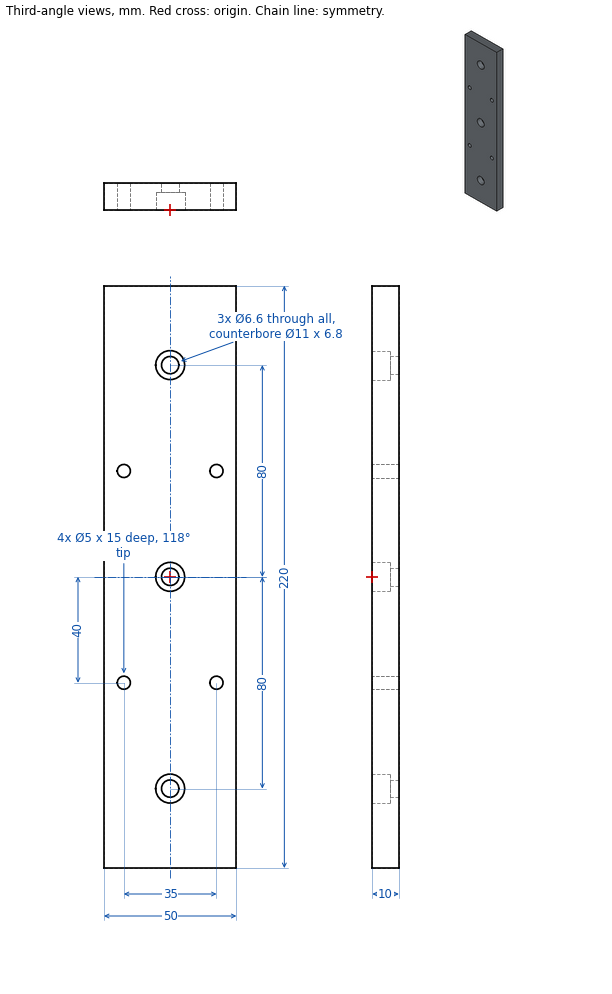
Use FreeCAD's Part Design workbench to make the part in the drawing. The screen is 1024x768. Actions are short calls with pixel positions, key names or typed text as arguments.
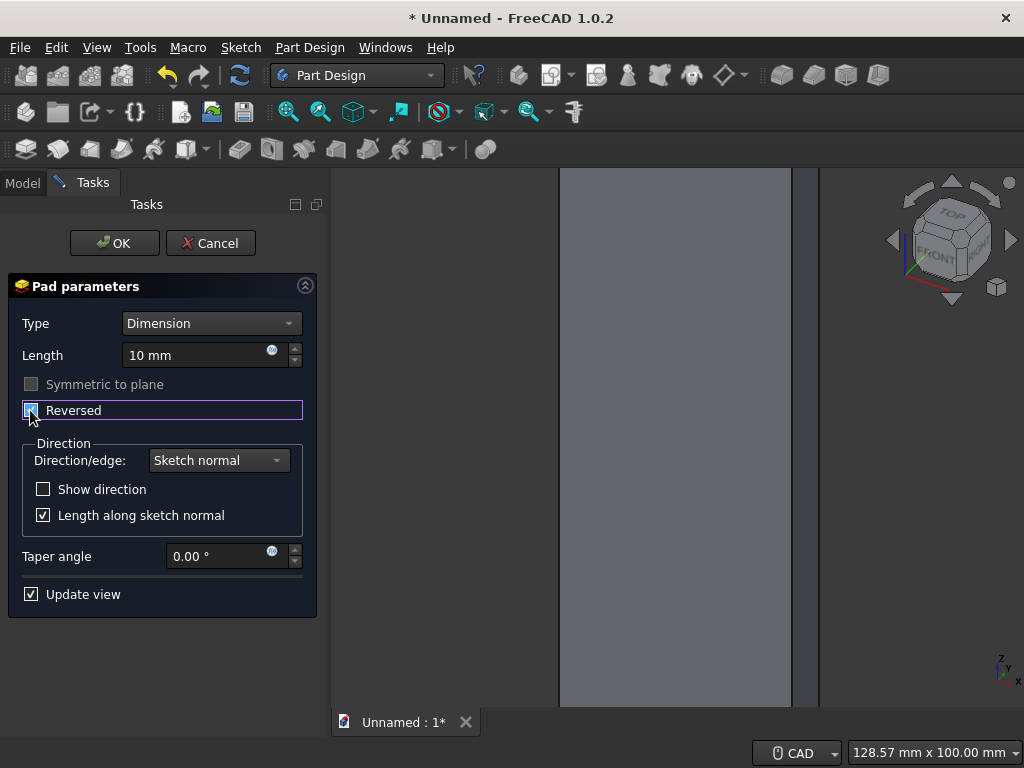
click(115, 243)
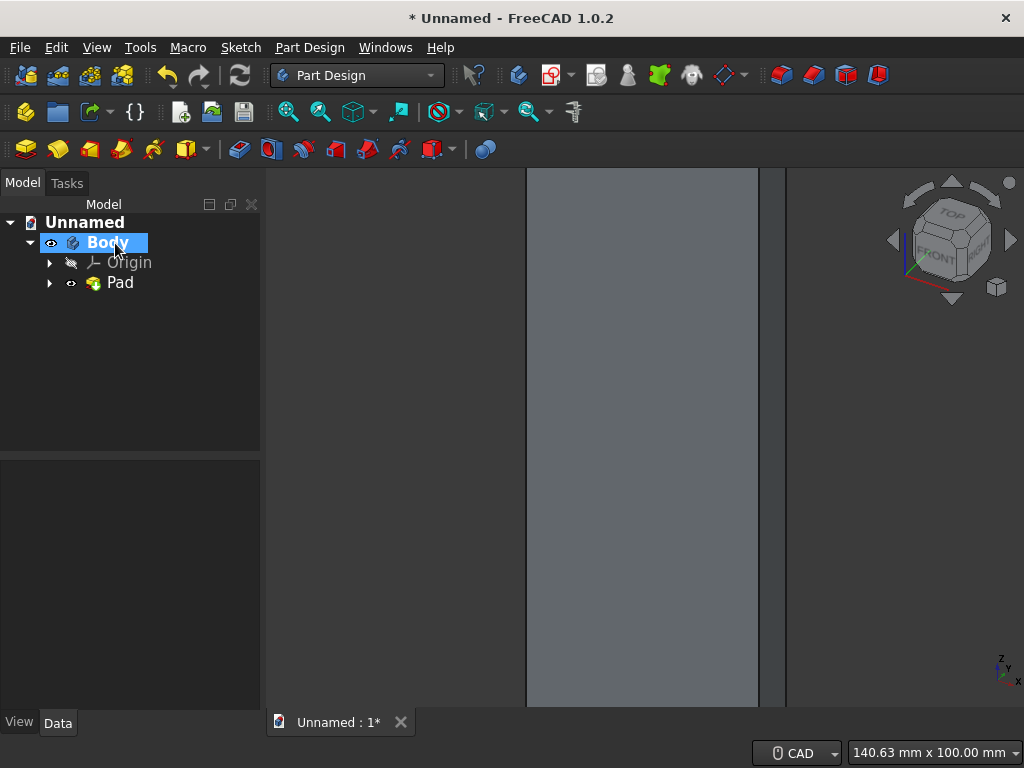
click(290, 112)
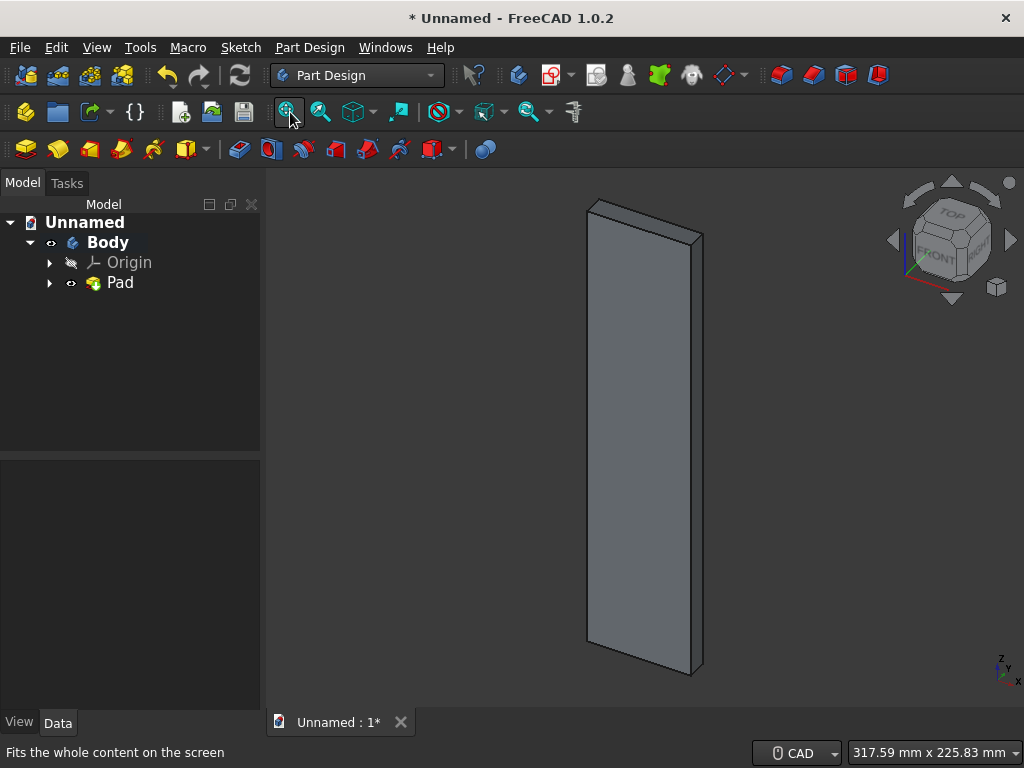
click(552, 76)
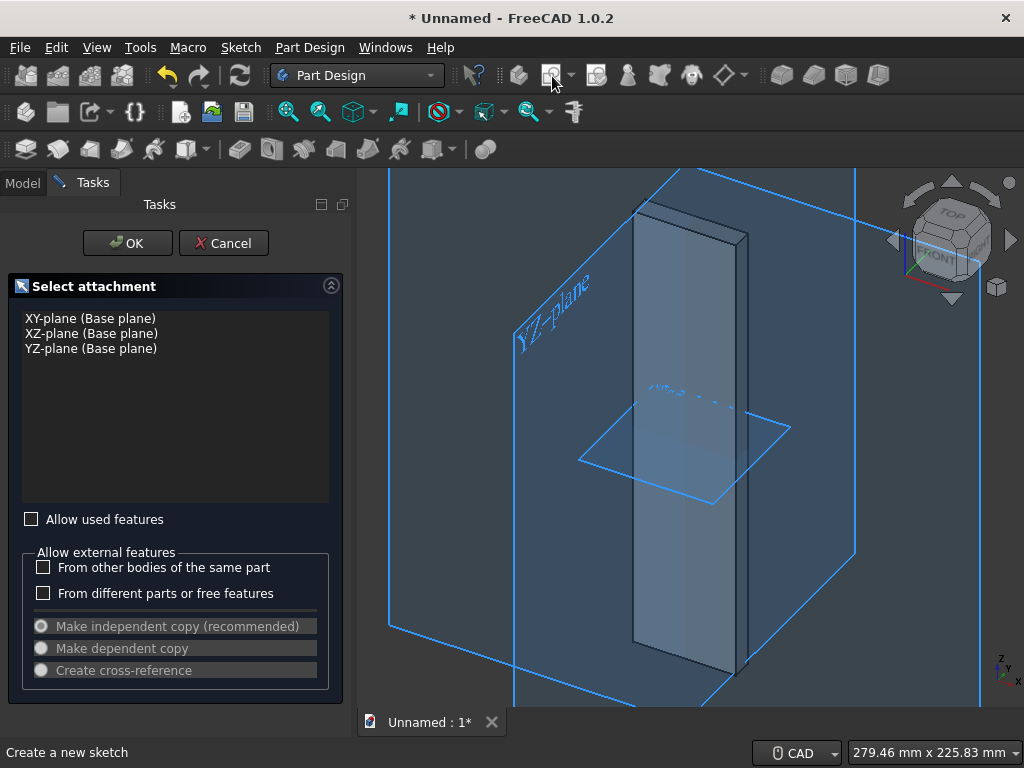
click(82, 334)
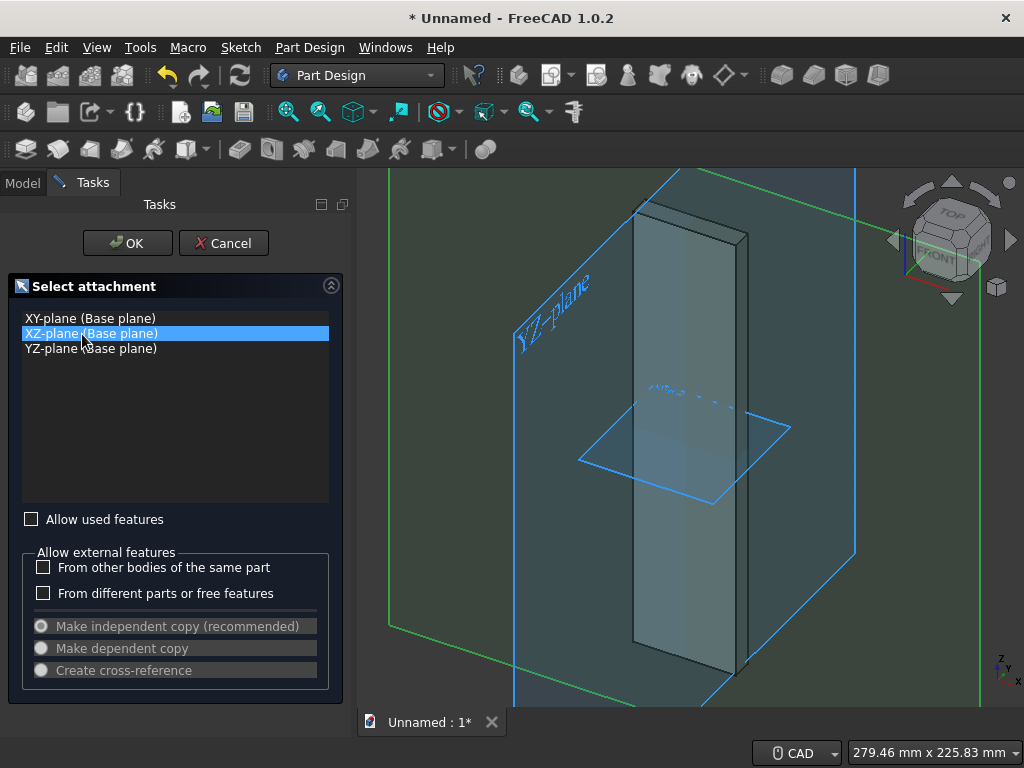
click(128, 243)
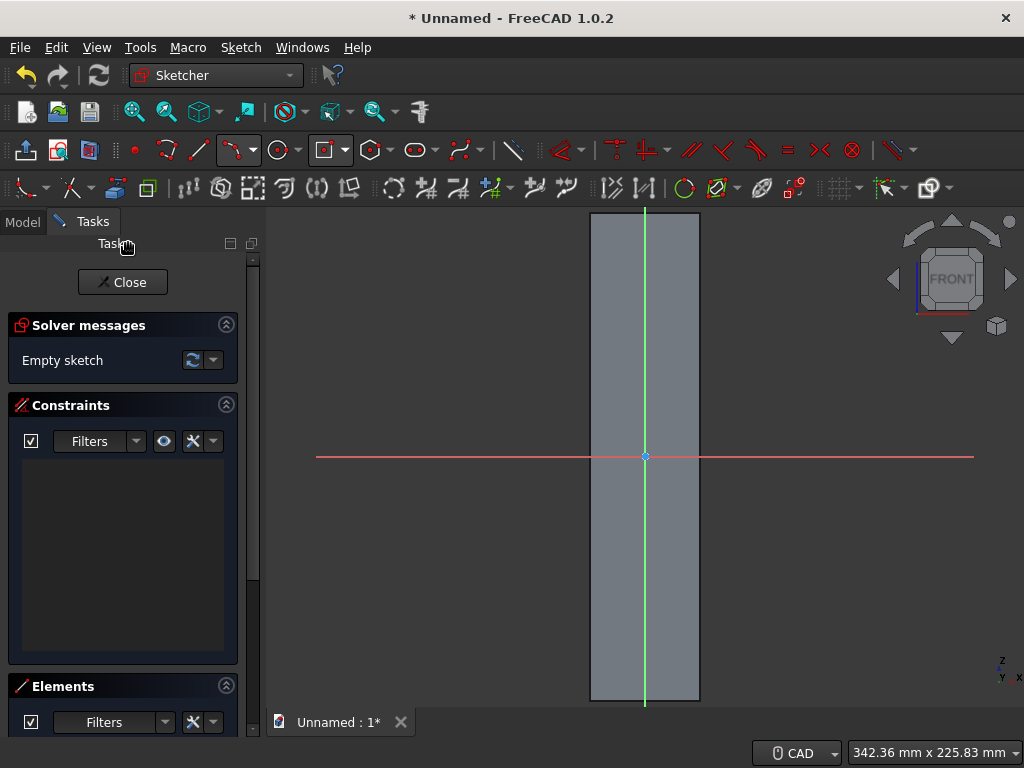
click(278, 150)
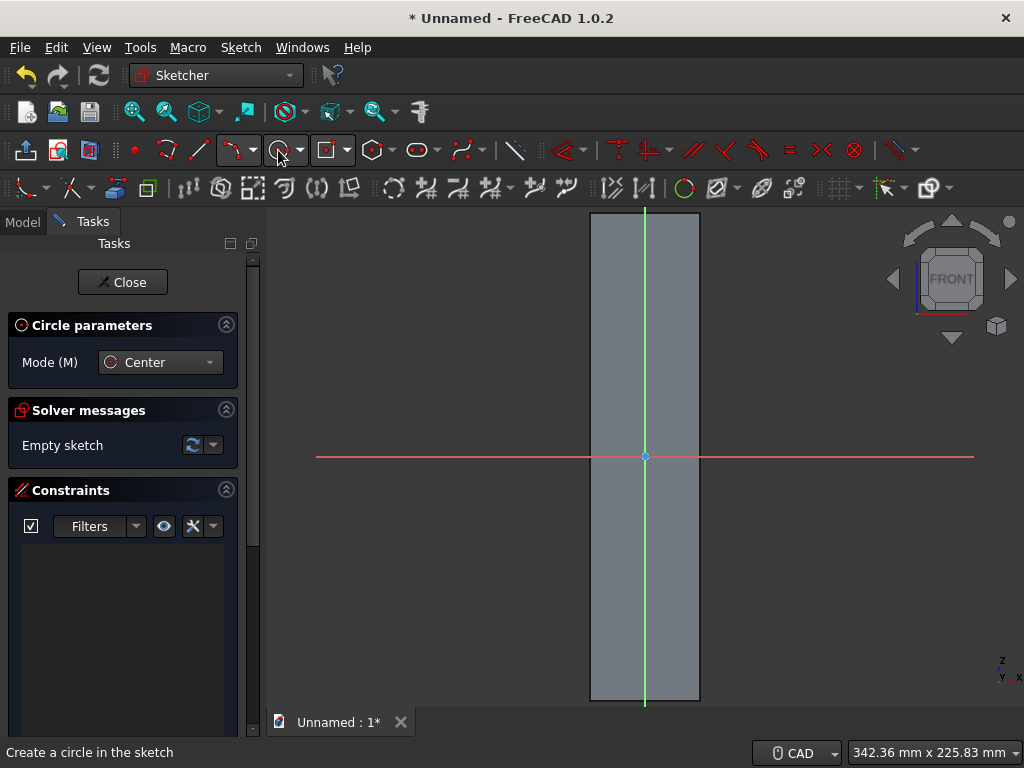
scroll(645, 280, up, 6)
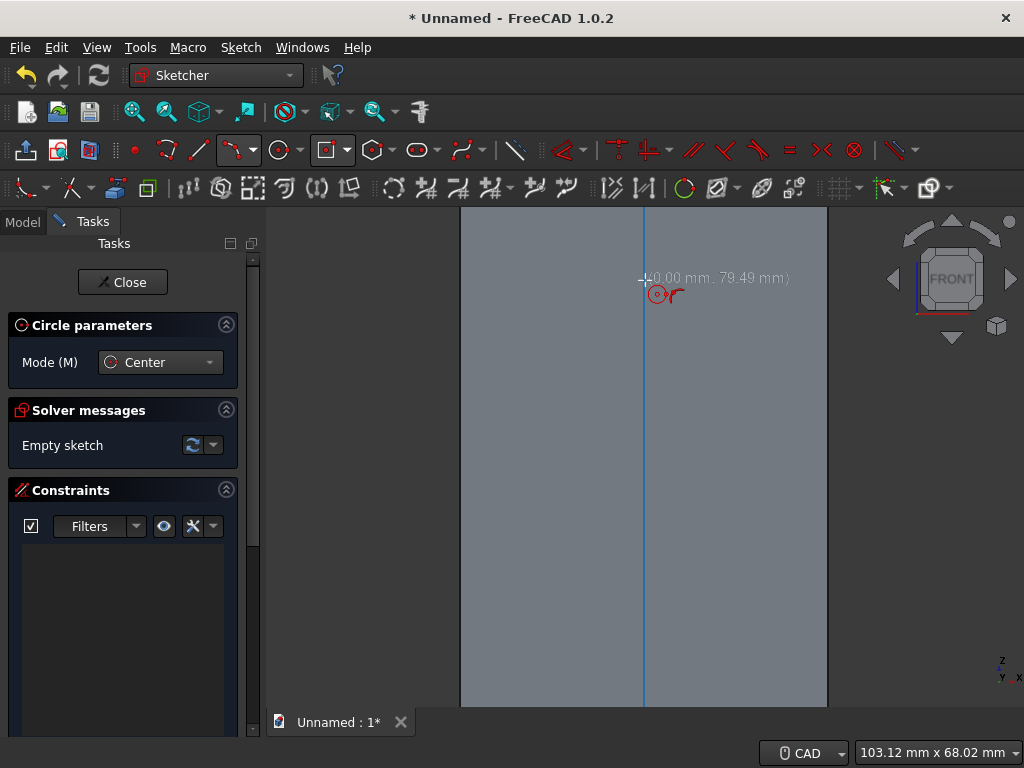
click(644, 279)
move(661, 262)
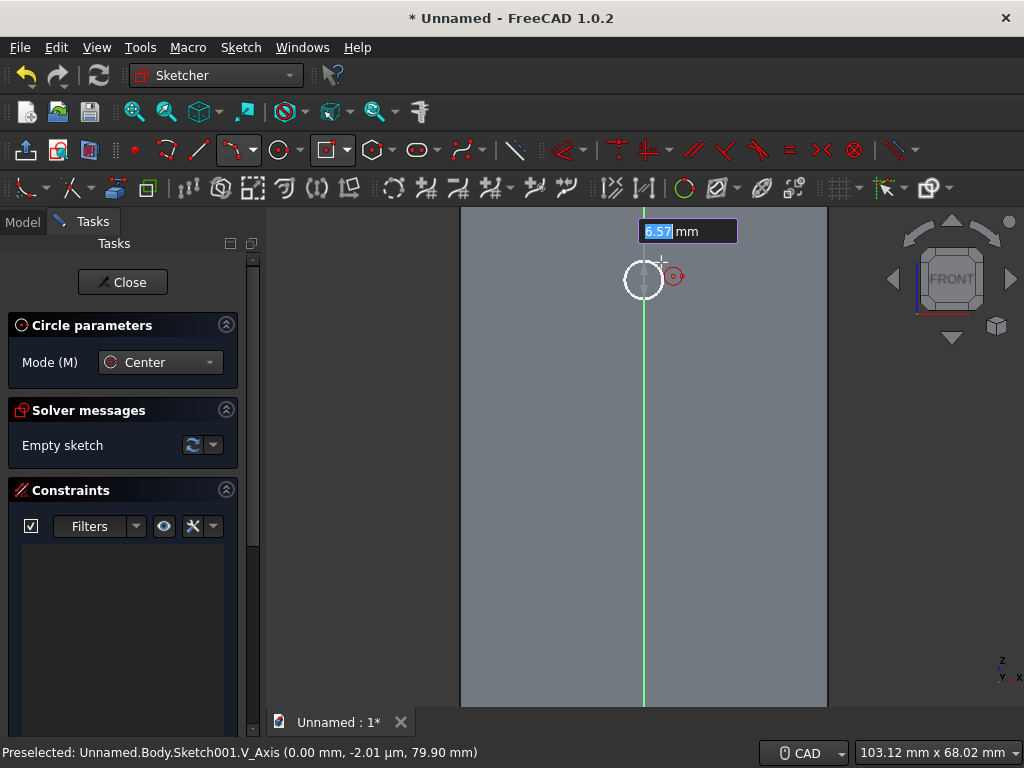
text(6.6)
key(Return)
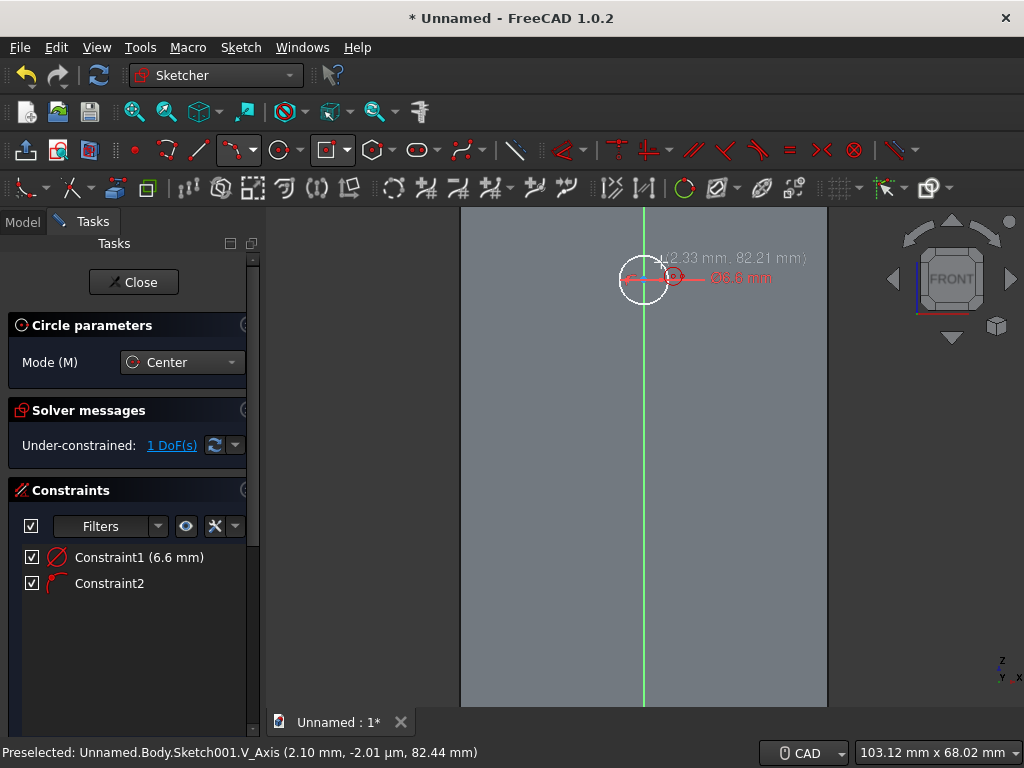
scroll(554, 323, down, 7)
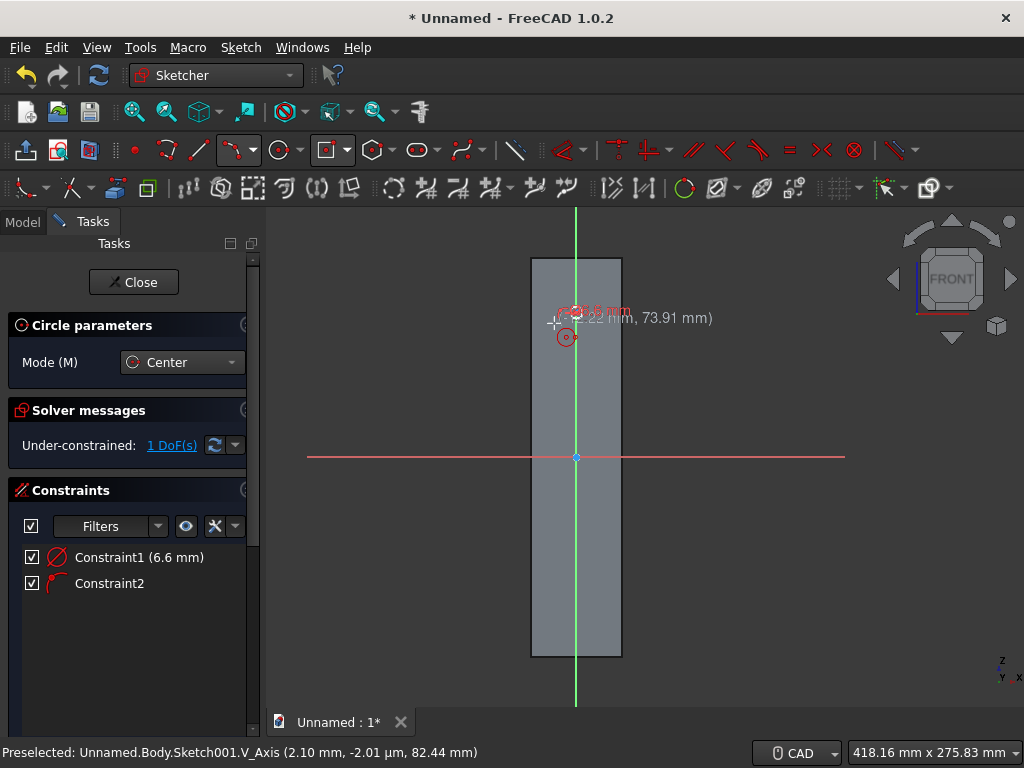
scroll(576, 602, up, 7)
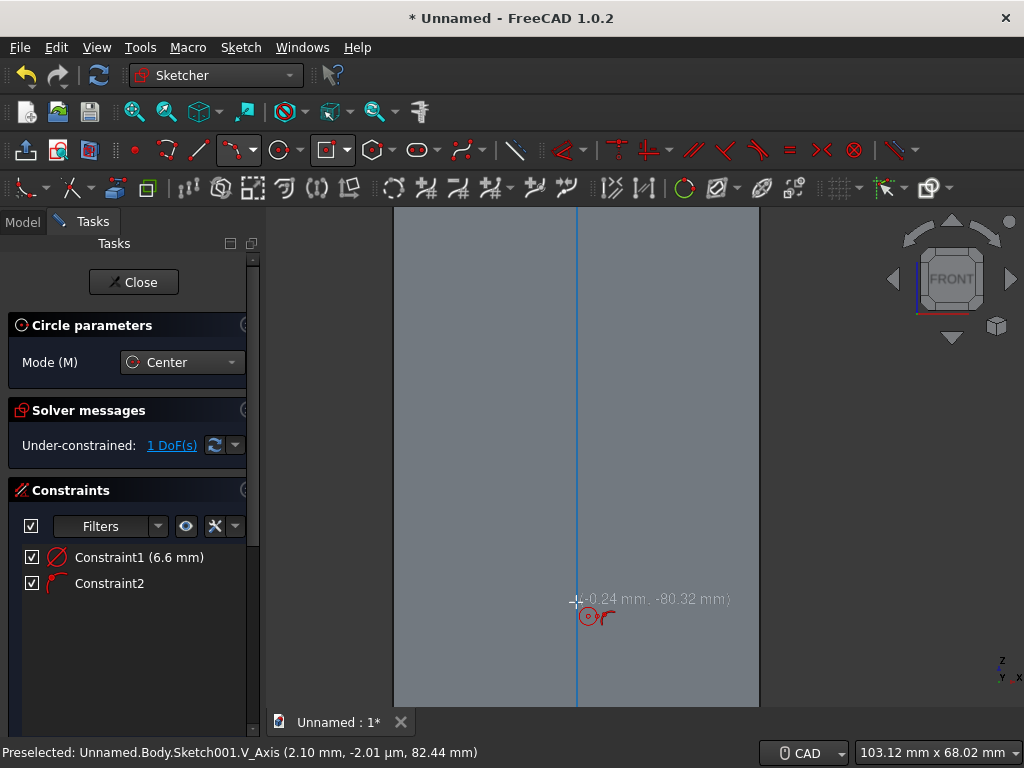
click(577, 601)
move(594, 584)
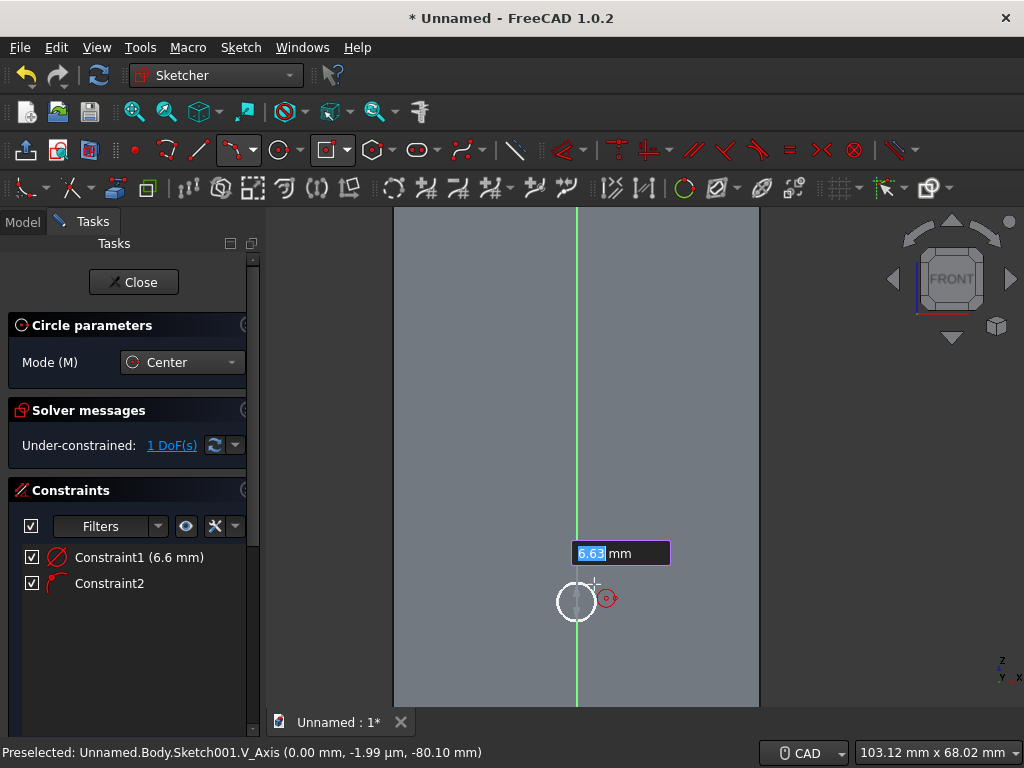
text(6.6)
key(Return)